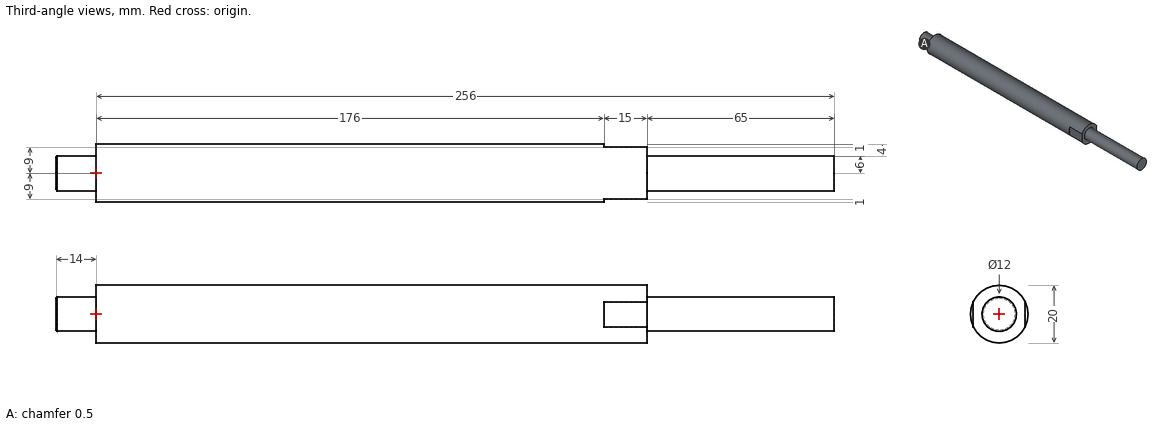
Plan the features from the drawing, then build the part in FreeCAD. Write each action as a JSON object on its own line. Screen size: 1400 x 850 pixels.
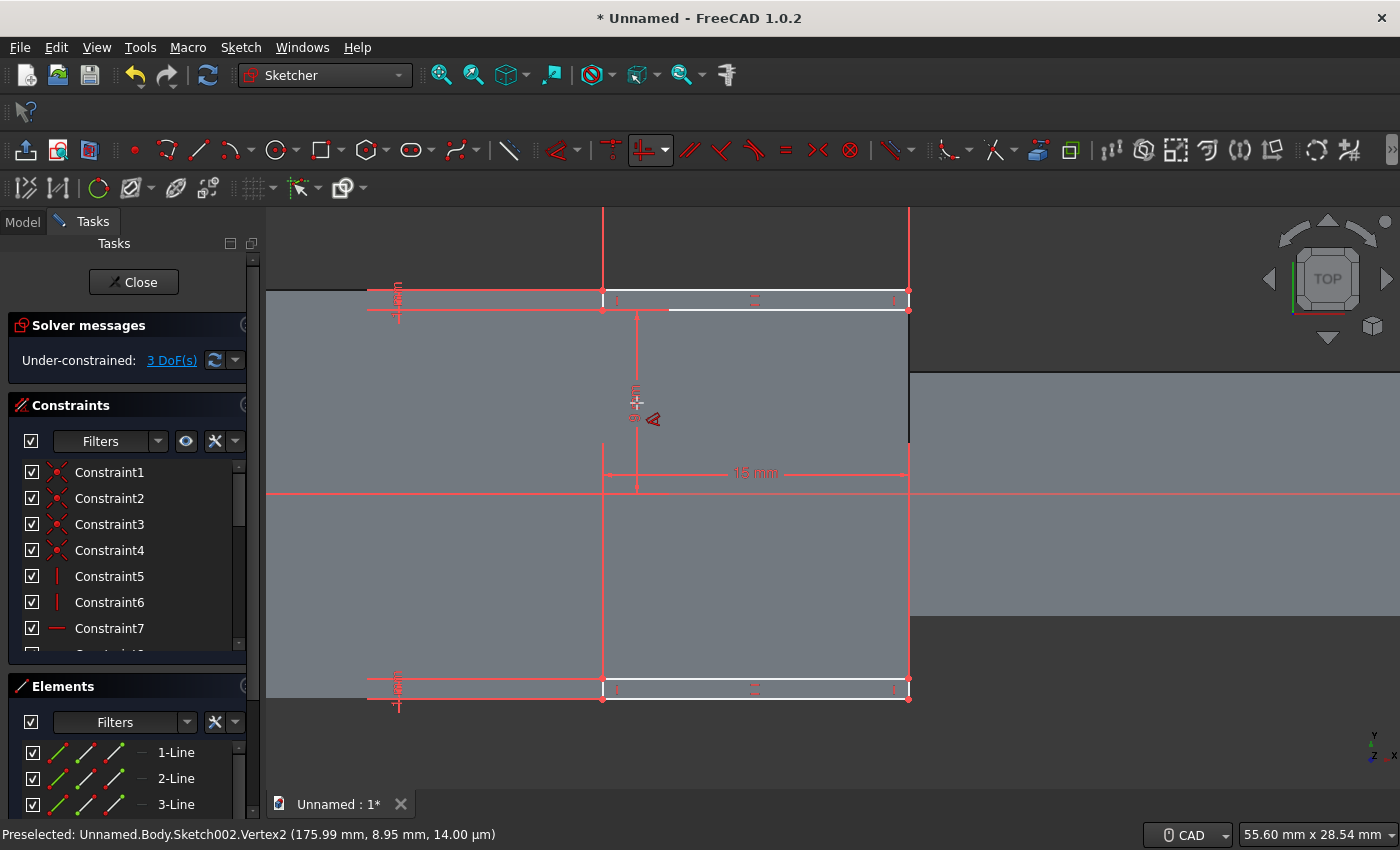
{"action": "left_click", "coordinate": [603, 679]}
{"action": "left_click", "coordinate": [637, 586]}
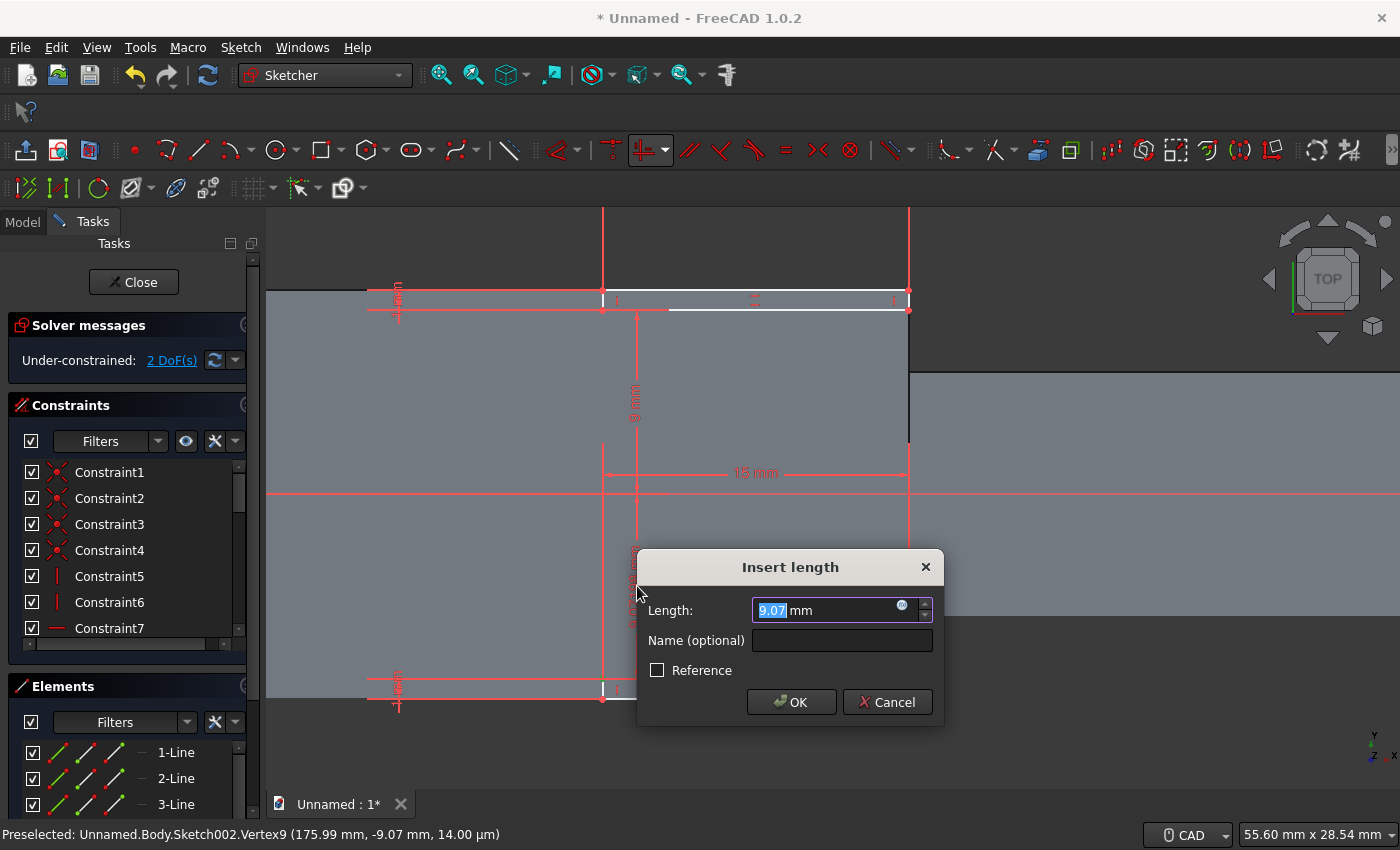
{"action": "type", "text": "9"}
{"action": "key", "text": "Return"}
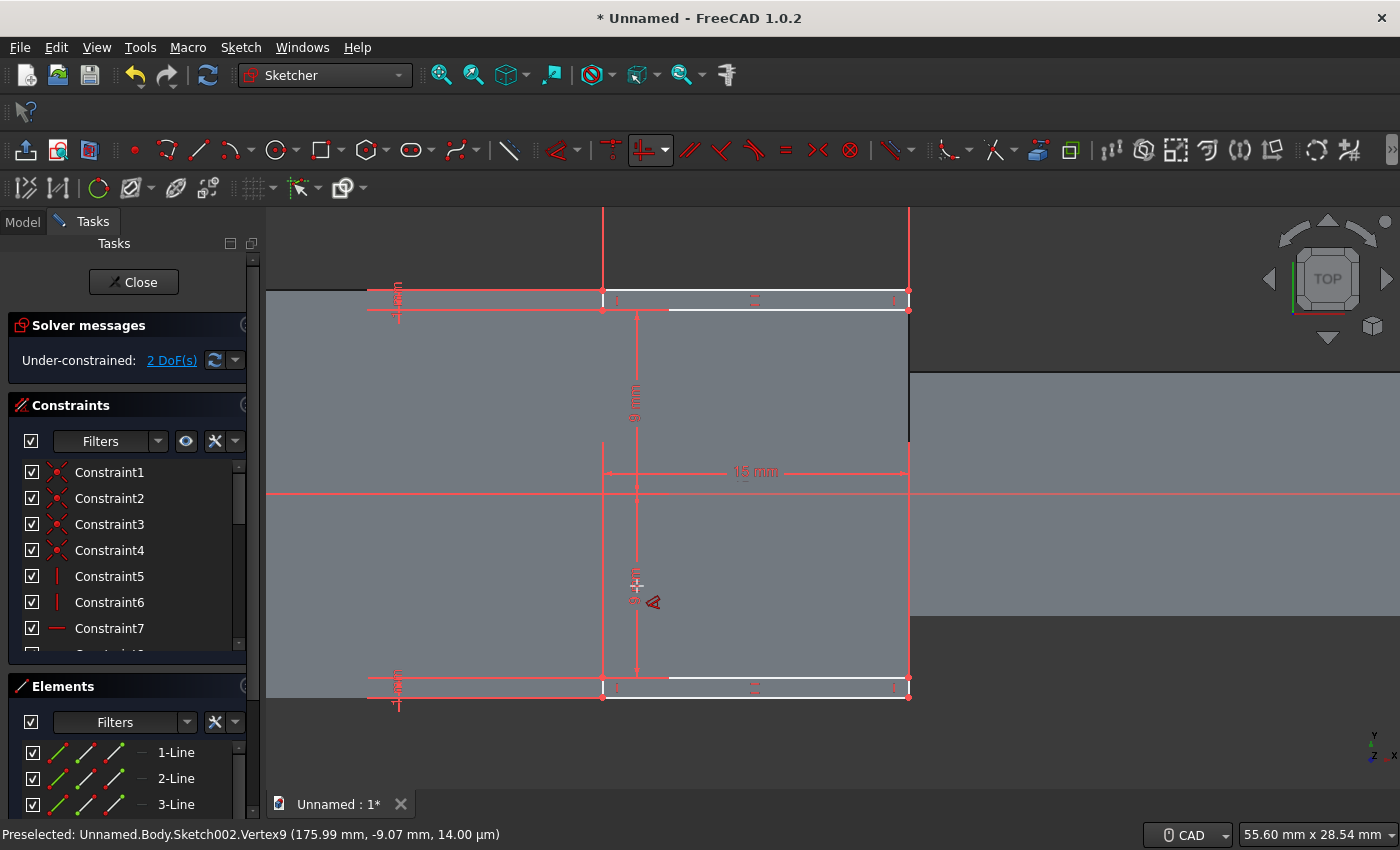
{"action": "left_click", "coordinate": [603, 290]}
{"action": "left_click", "coordinate": [449, 256]}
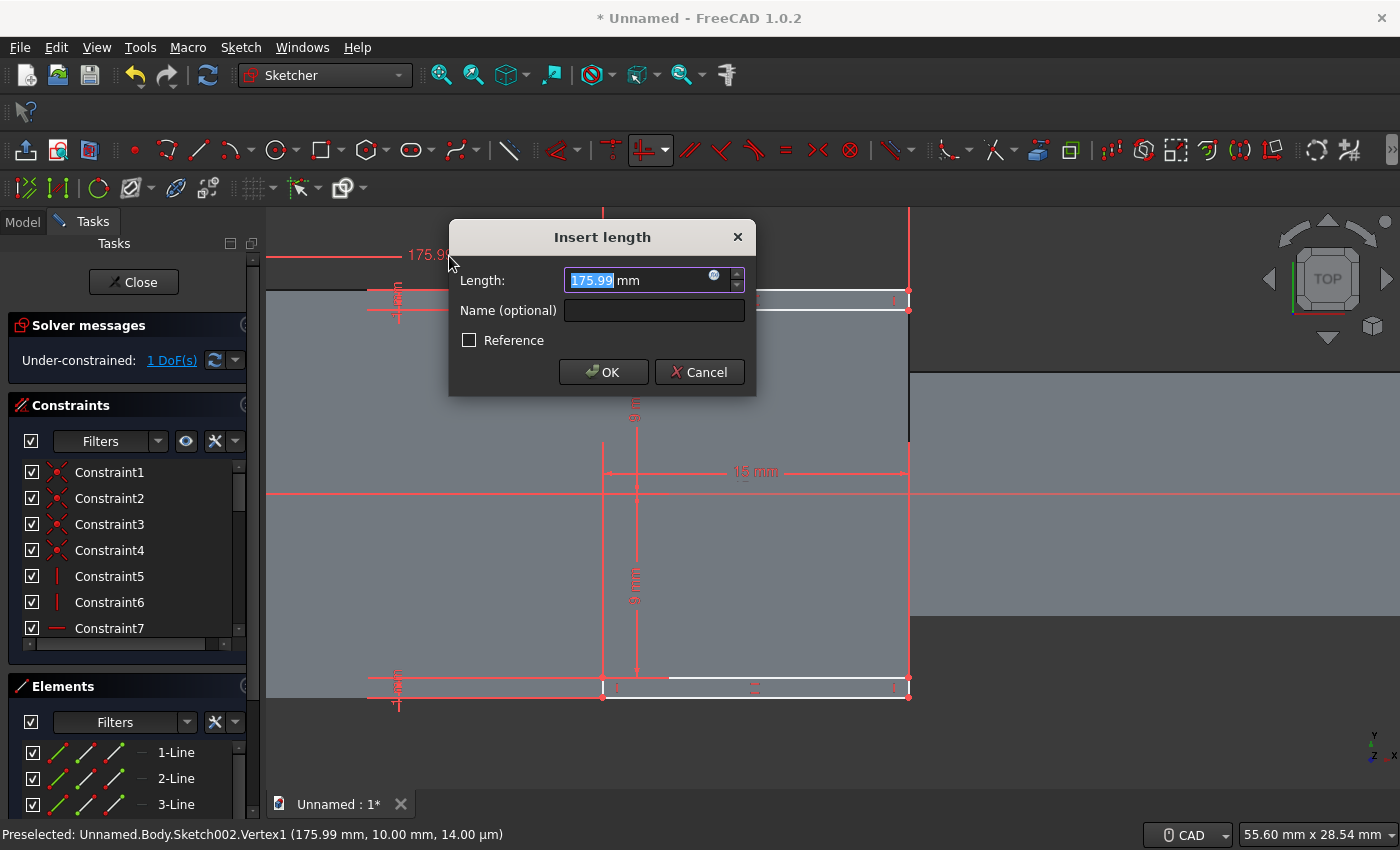
{"action": "type", "text": "176"}
{"action": "key", "text": "Return"}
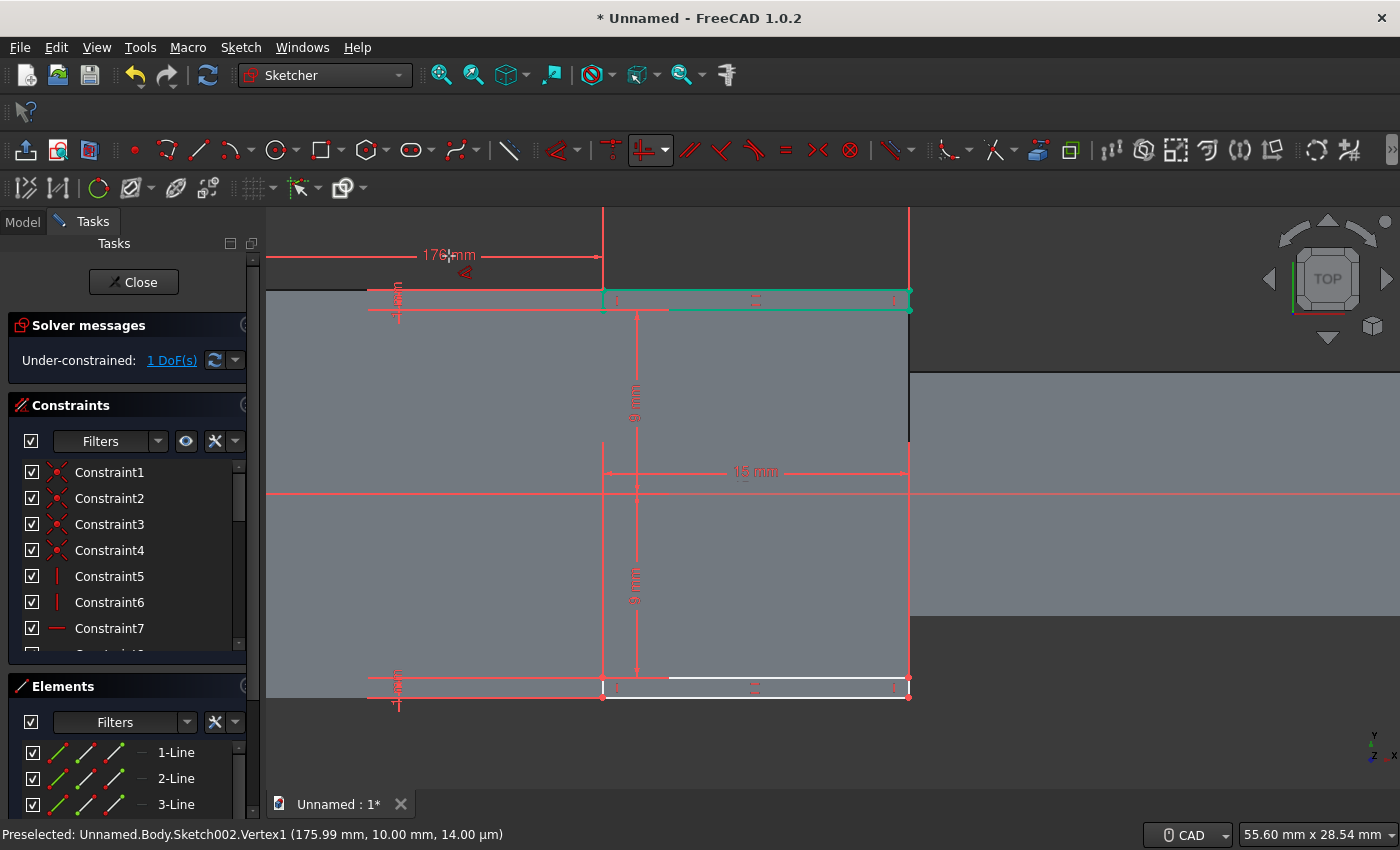
{"action": "left_click", "coordinate": [603, 678]}
{"action": "left_click", "coordinate": [449, 712]}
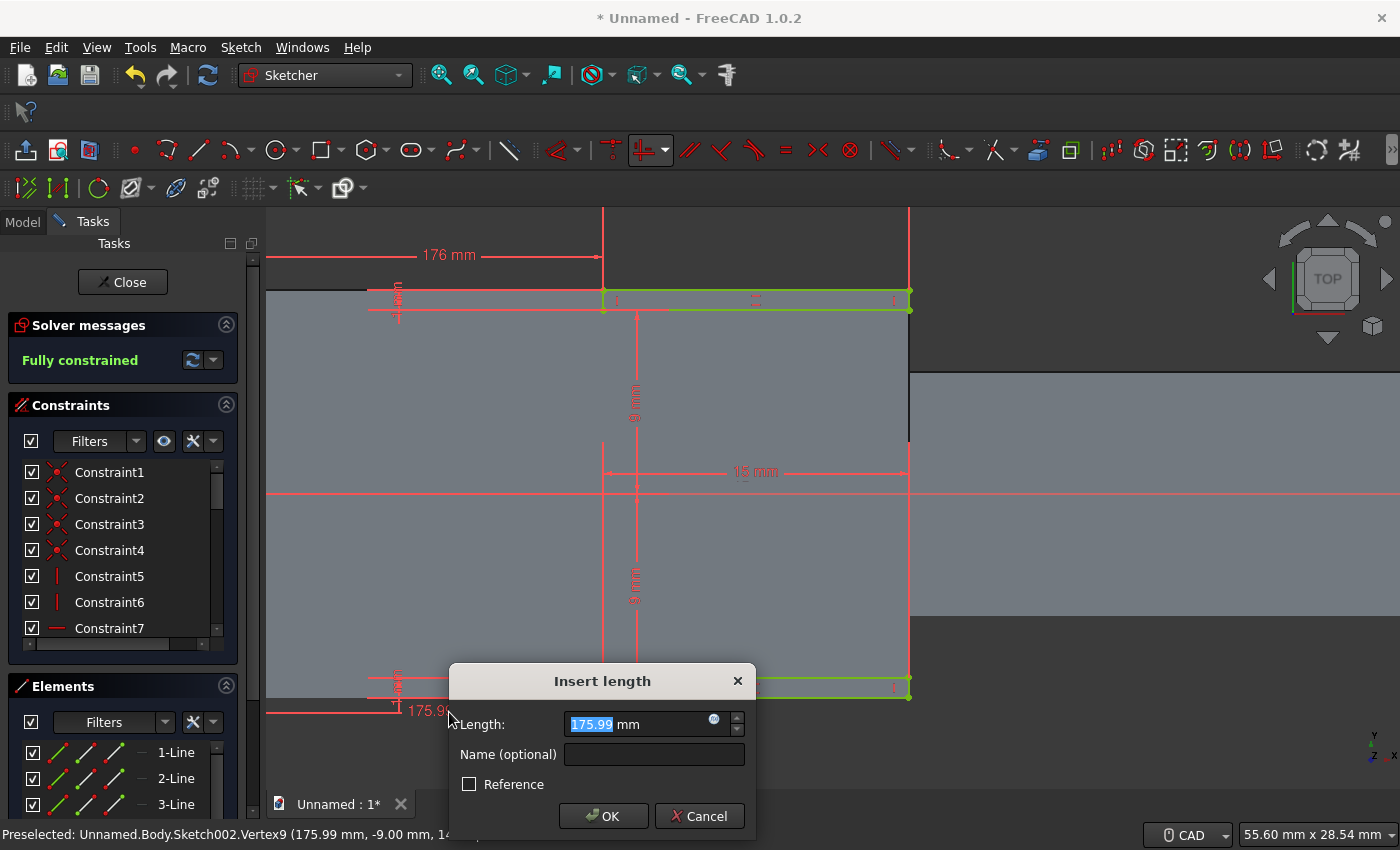
{"action": "type", "text": "176"}
{"action": "key", "text": "Return"}
{"action": "key", "text": "Escape"}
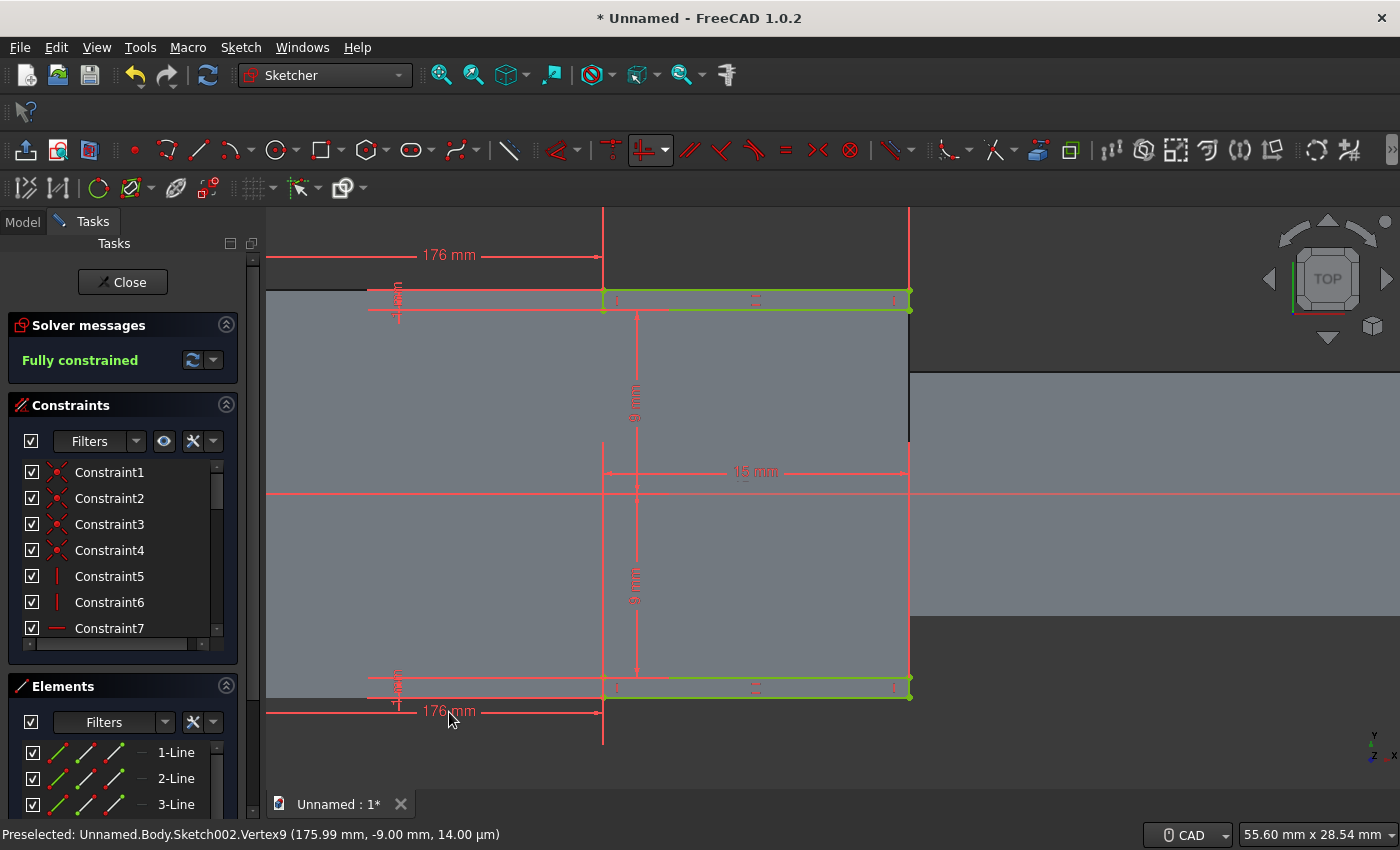
{"action": "left_click", "coordinate": [123, 282]}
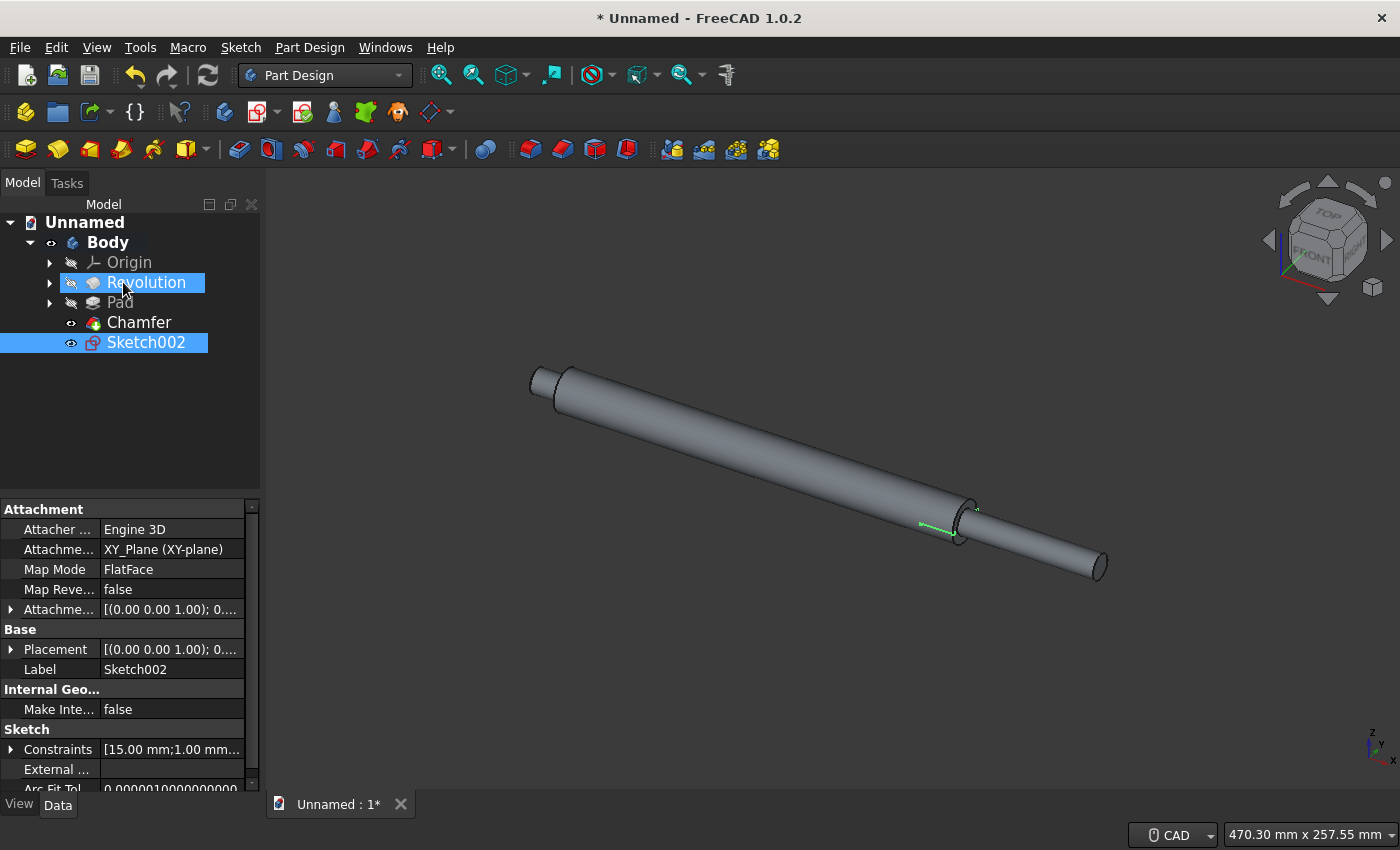
{"action": "left_click", "coordinate": [240, 150]}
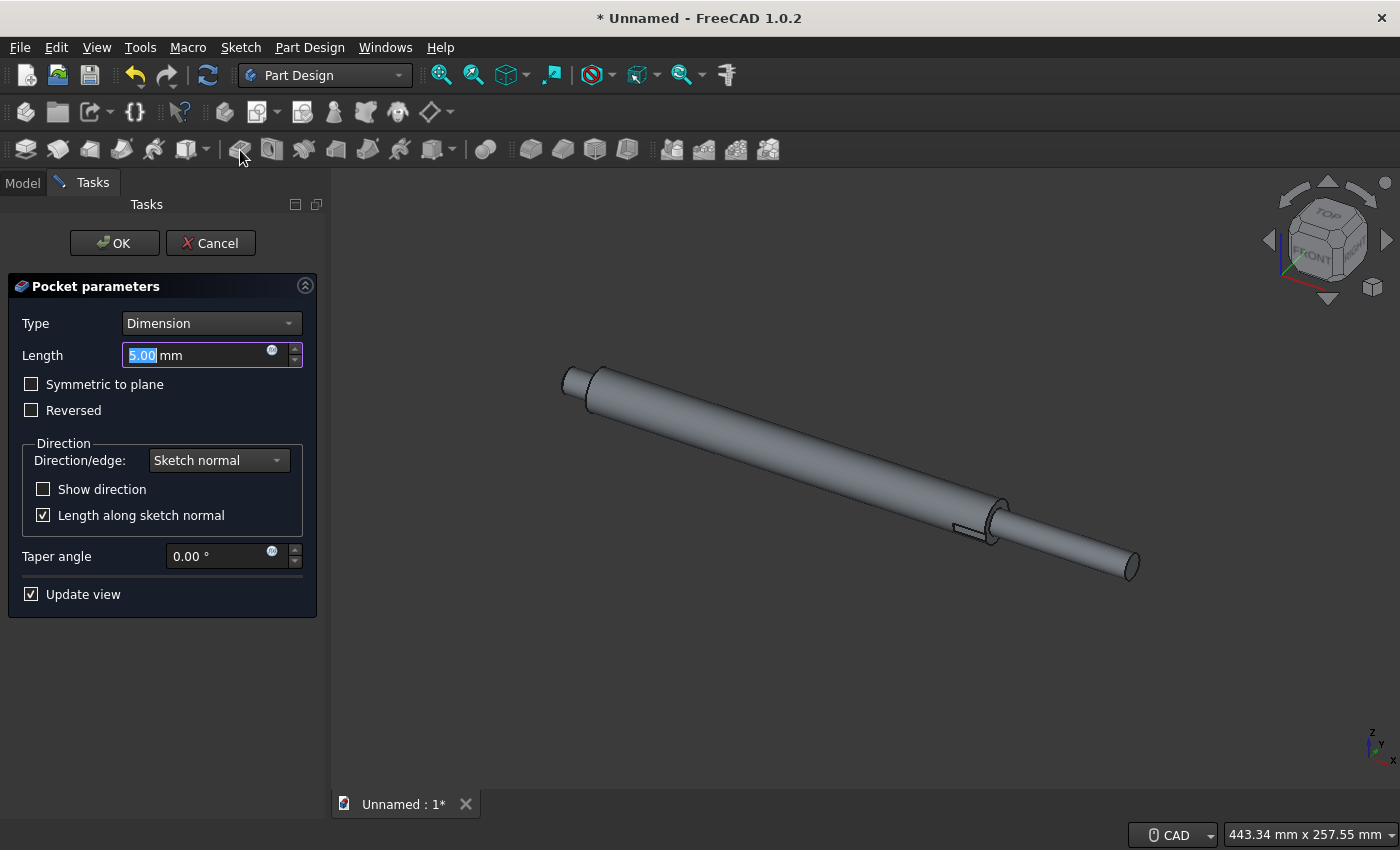
{"action": "type", "text": "20"}
{"action": "key", "text": "Tab"}